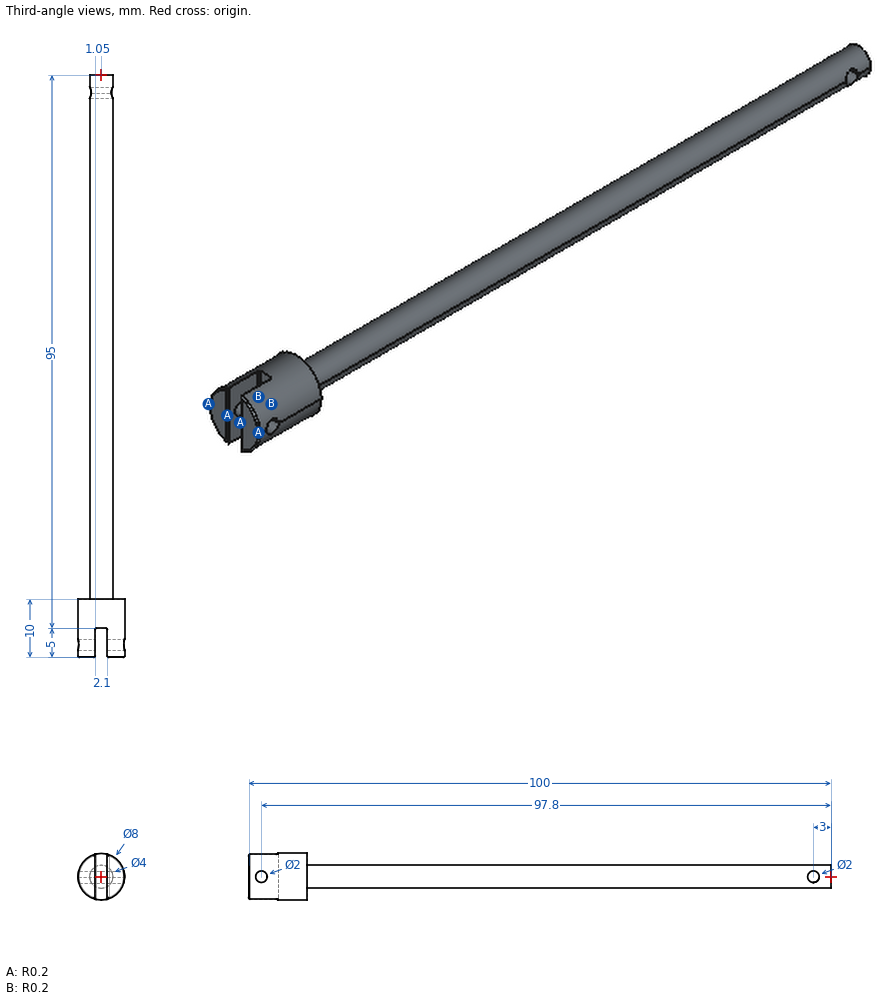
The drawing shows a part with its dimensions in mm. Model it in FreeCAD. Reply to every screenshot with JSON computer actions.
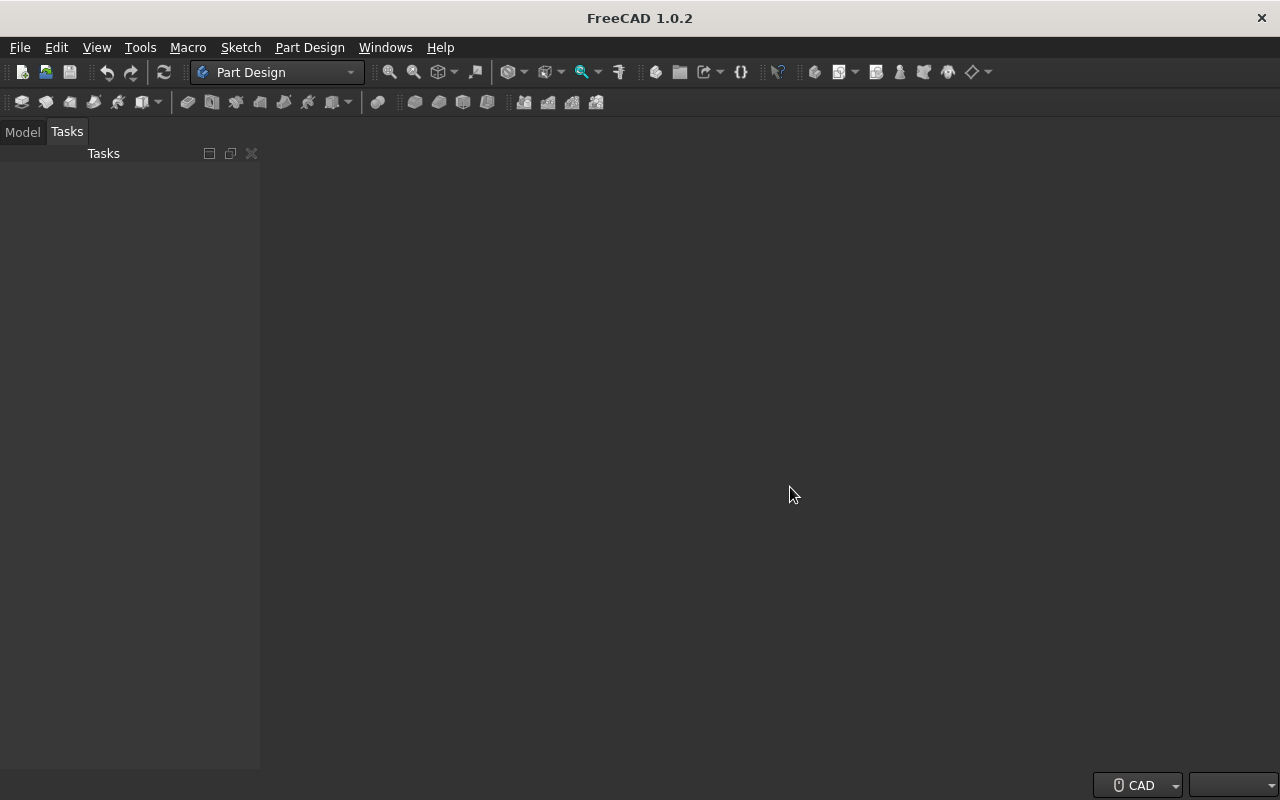
{"action": "left_click", "coordinate": [22, 72]}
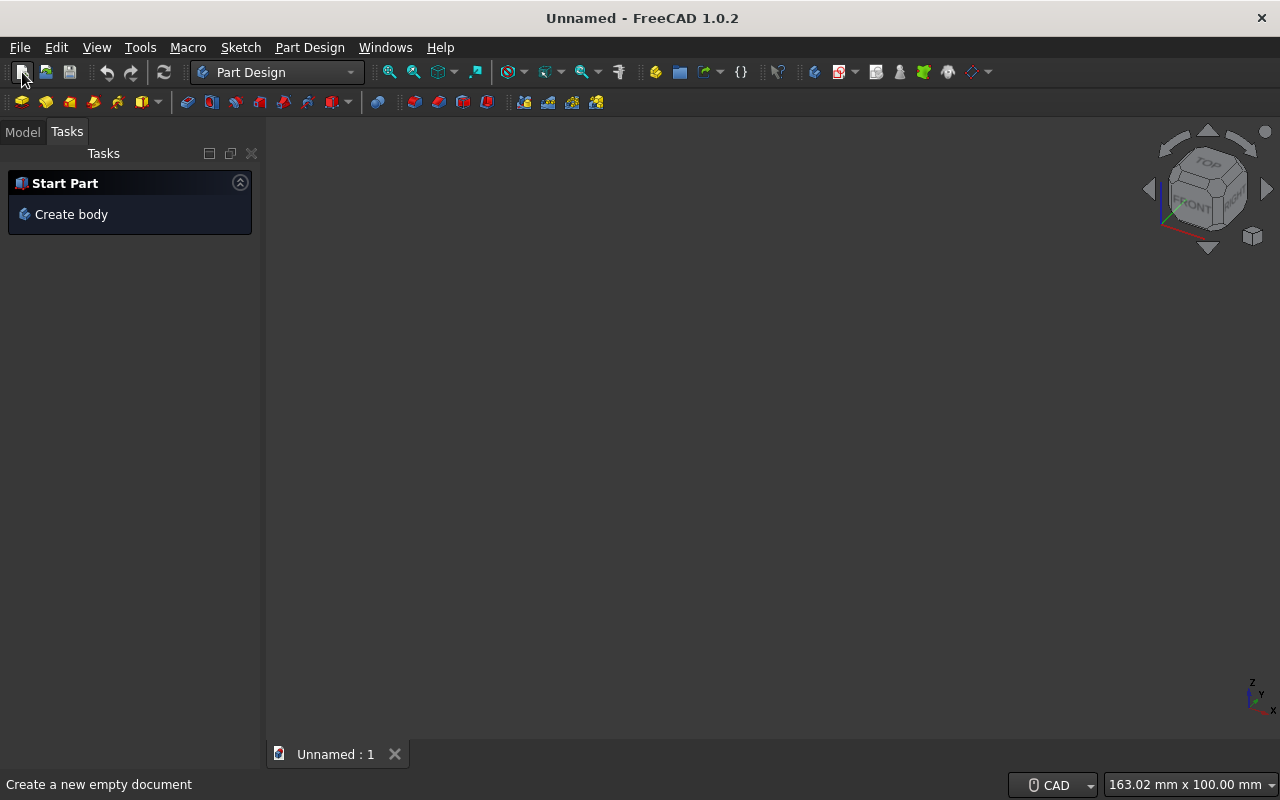
{"action": "left_click", "coordinate": [840, 72]}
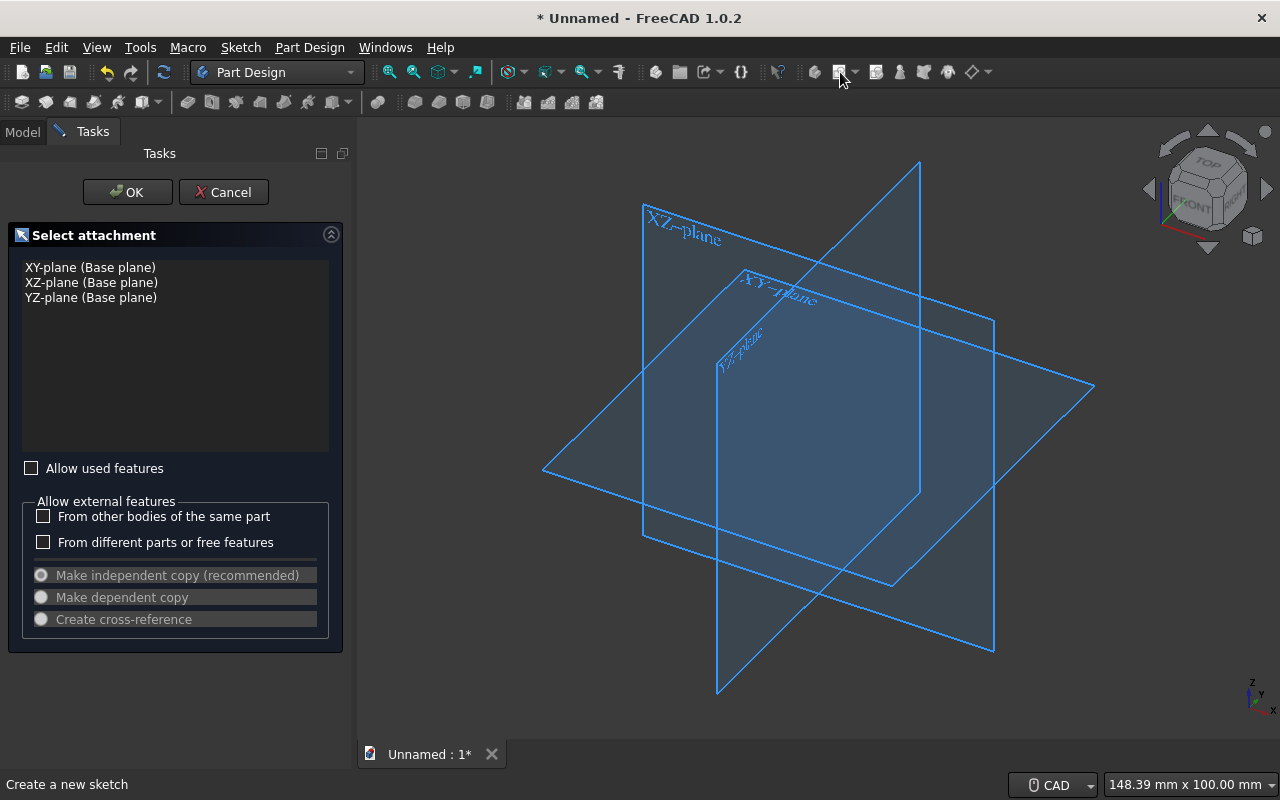
{"action": "left_click", "coordinate": [82, 282]}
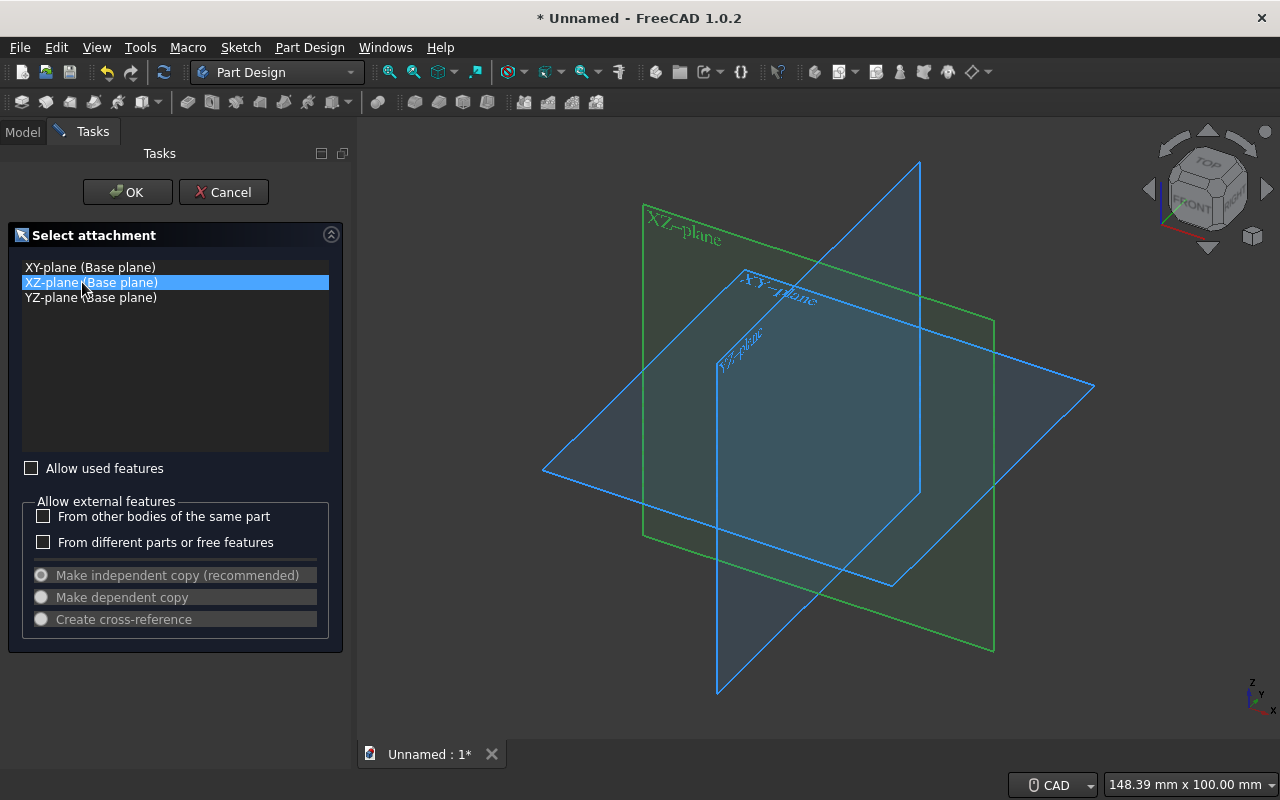
{"action": "left_click", "coordinate": [128, 192]}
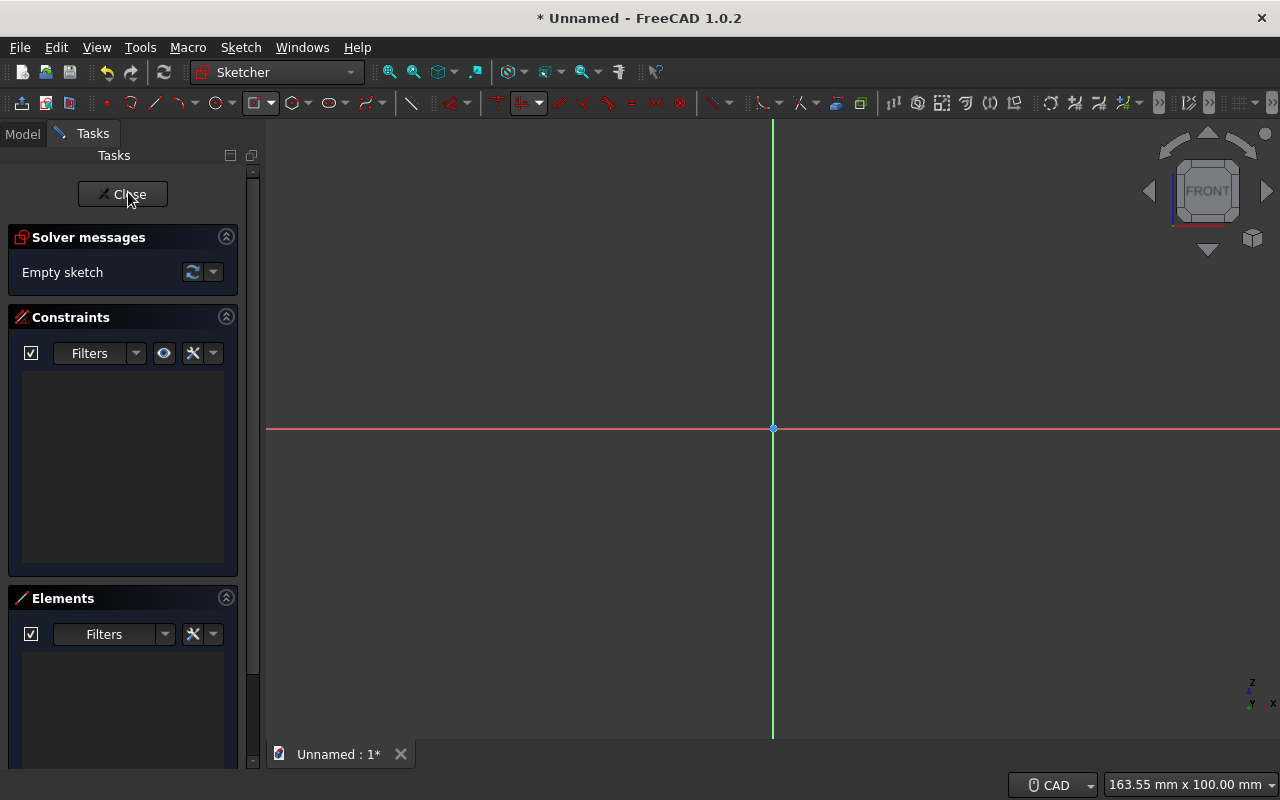
{"action": "scroll", "coordinate": [777, 429], "scroll_direction": "up", "scroll_amount": 14}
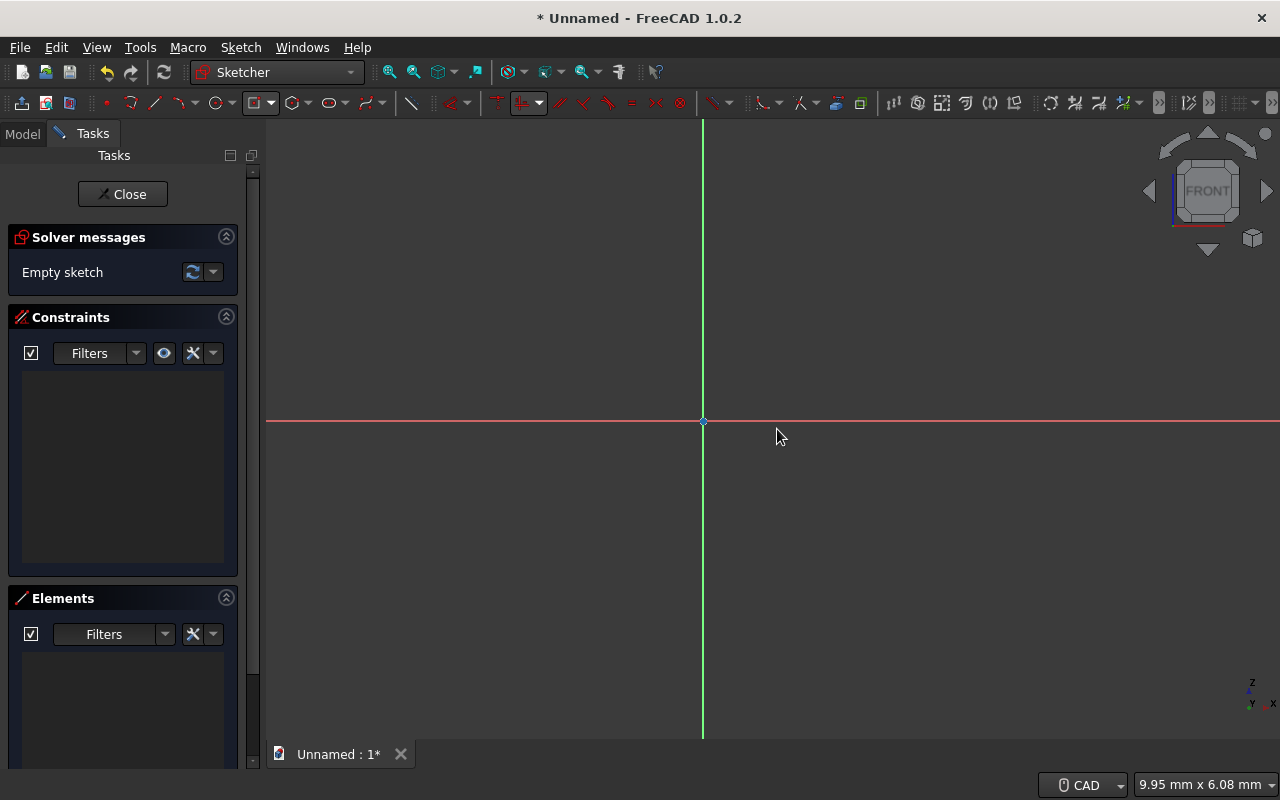
{"action": "left_click", "coordinate": [216, 104]}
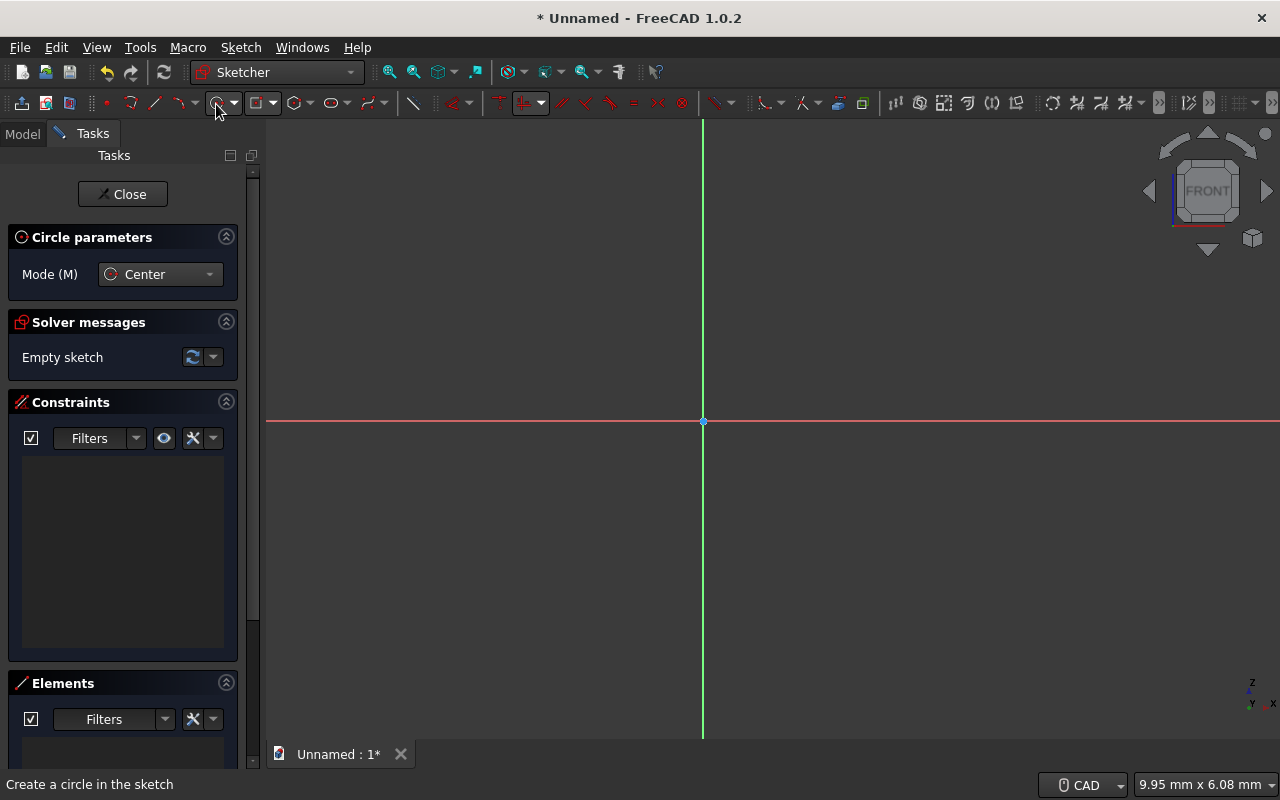
{"action": "left_click", "coordinate": [703, 421]}
{"action": "left_click", "coordinate": [848, 277]}
{"action": "key", "text": "Escape"}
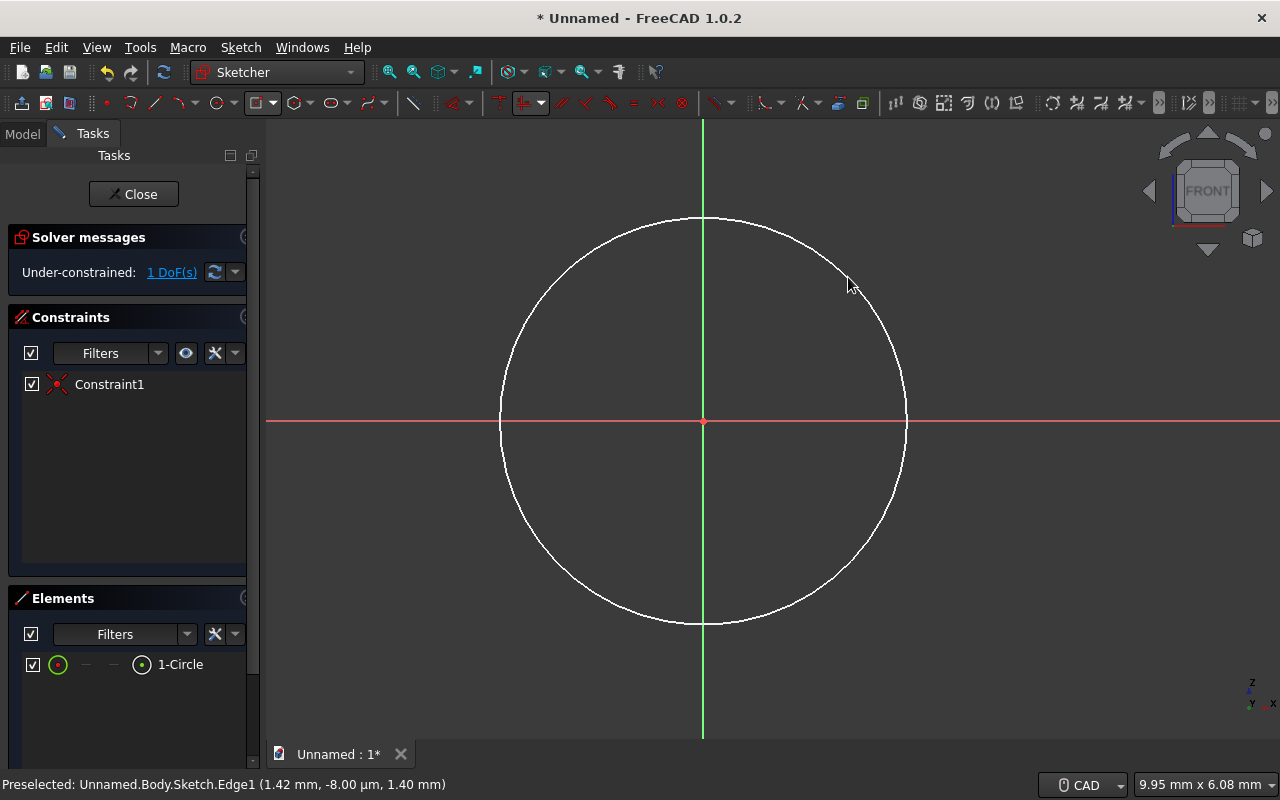
{"action": "left_click", "coordinate": [452, 104]}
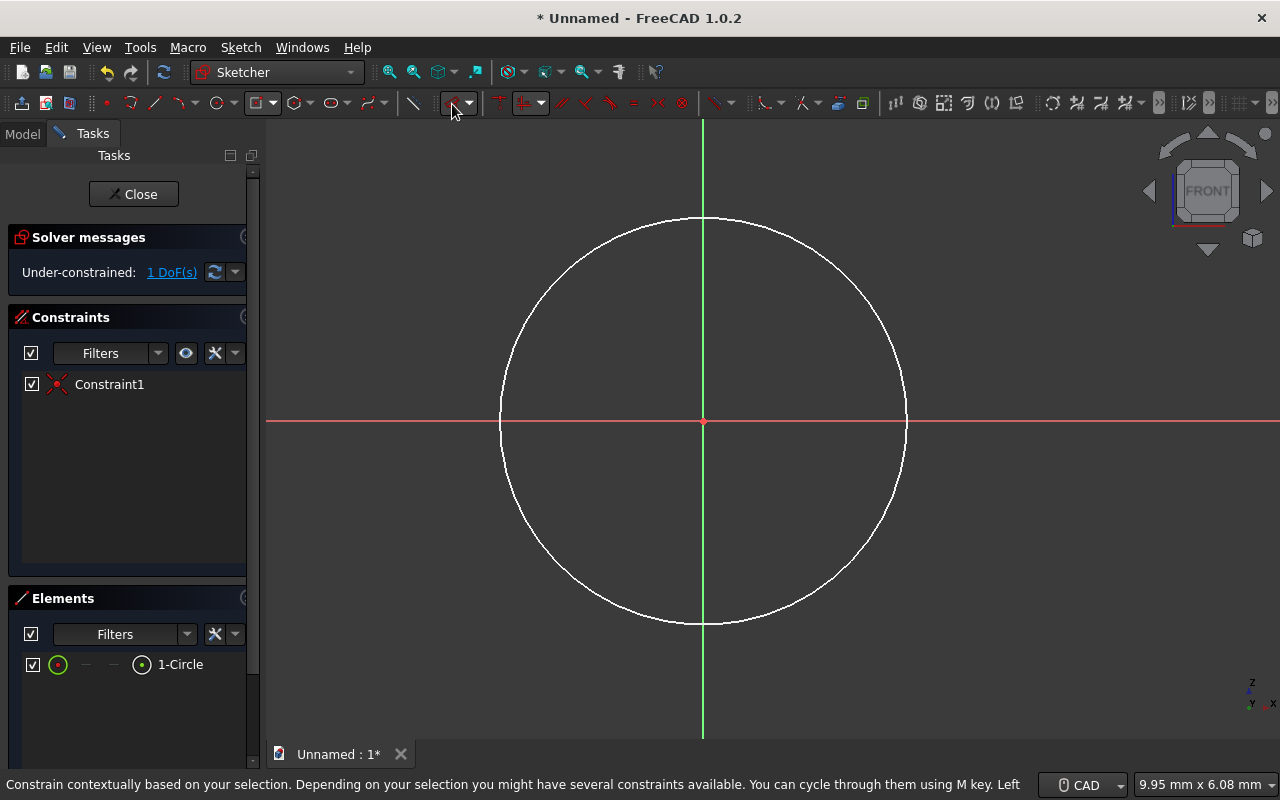
{"action": "left_click", "coordinate": [847, 277]}
{"action": "left_click", "coordinate": [870, 254]}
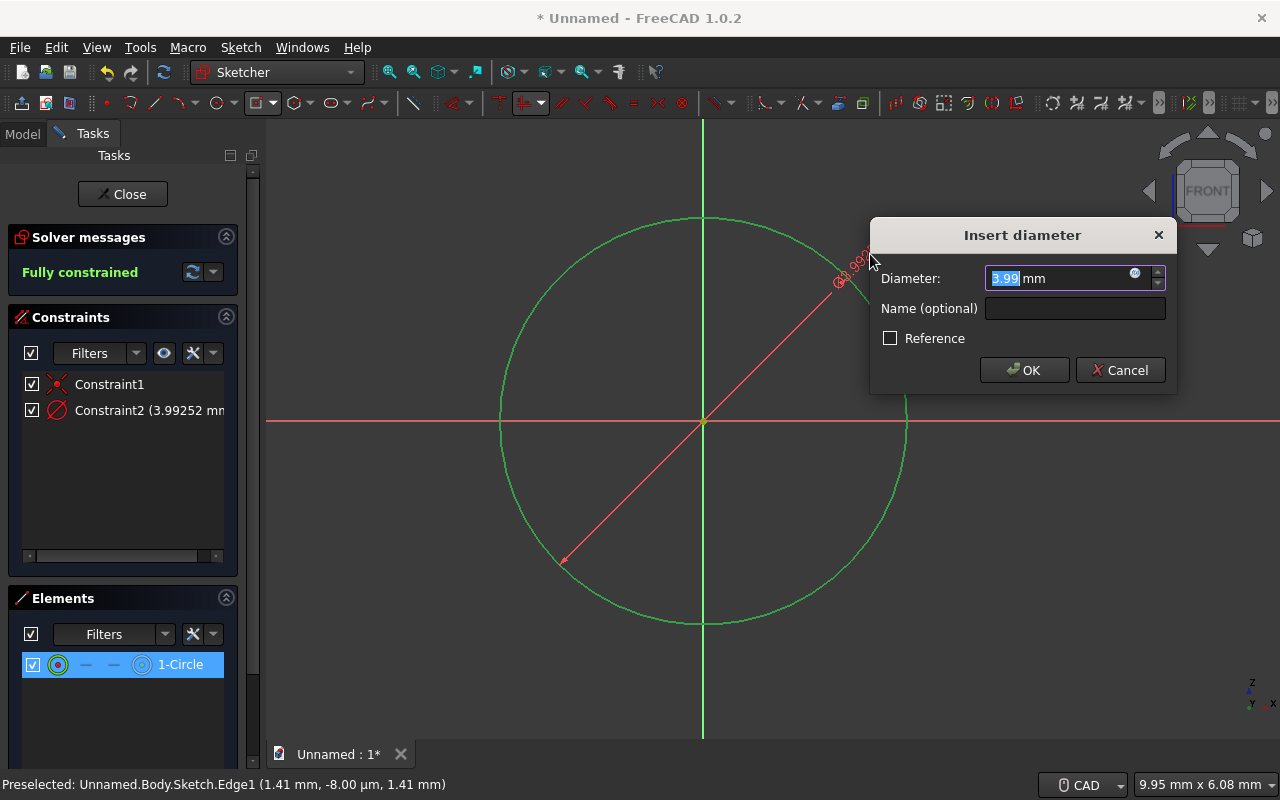
{"action": "type", "text": "4"}
{"action": "key", "text": "Return"}
{"action": "key", "text": "Escape"}